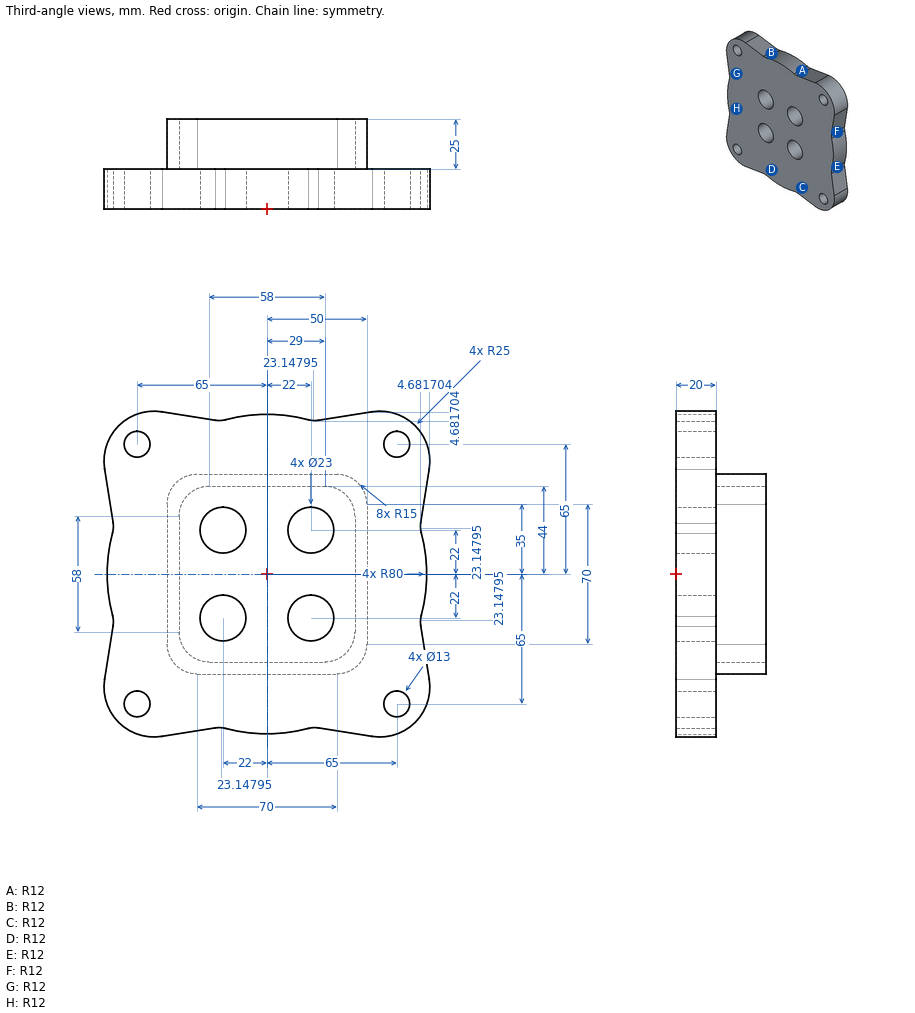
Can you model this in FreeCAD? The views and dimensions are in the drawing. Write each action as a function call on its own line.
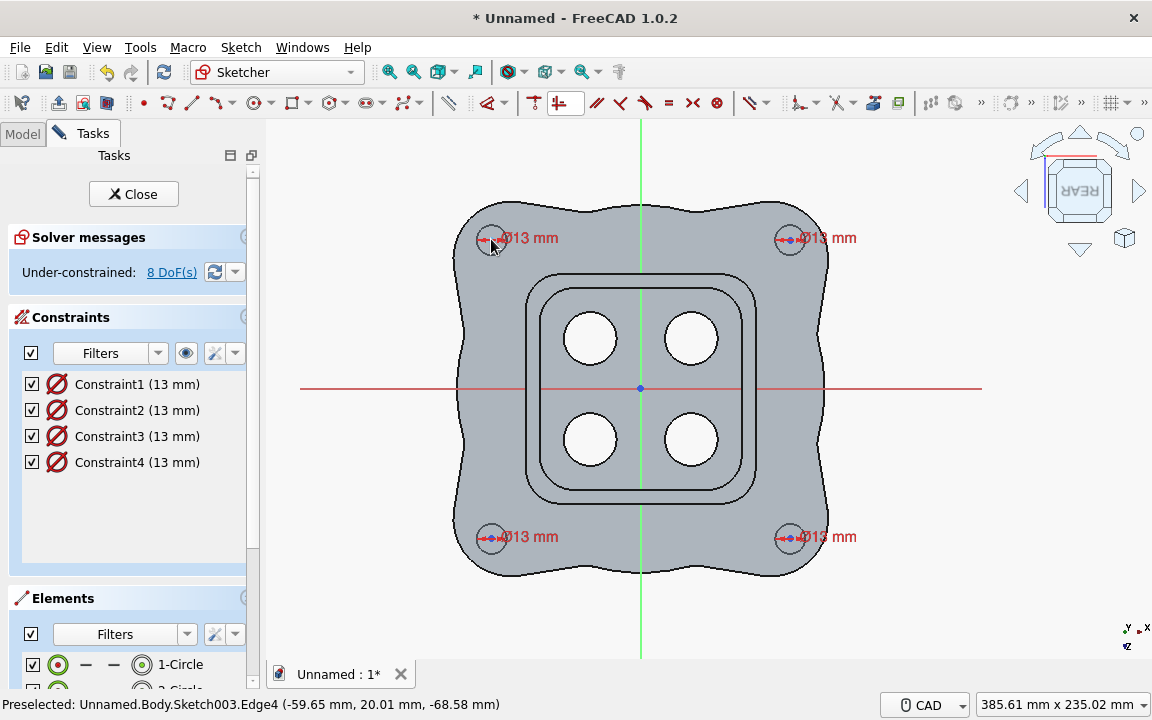
click(790, 240)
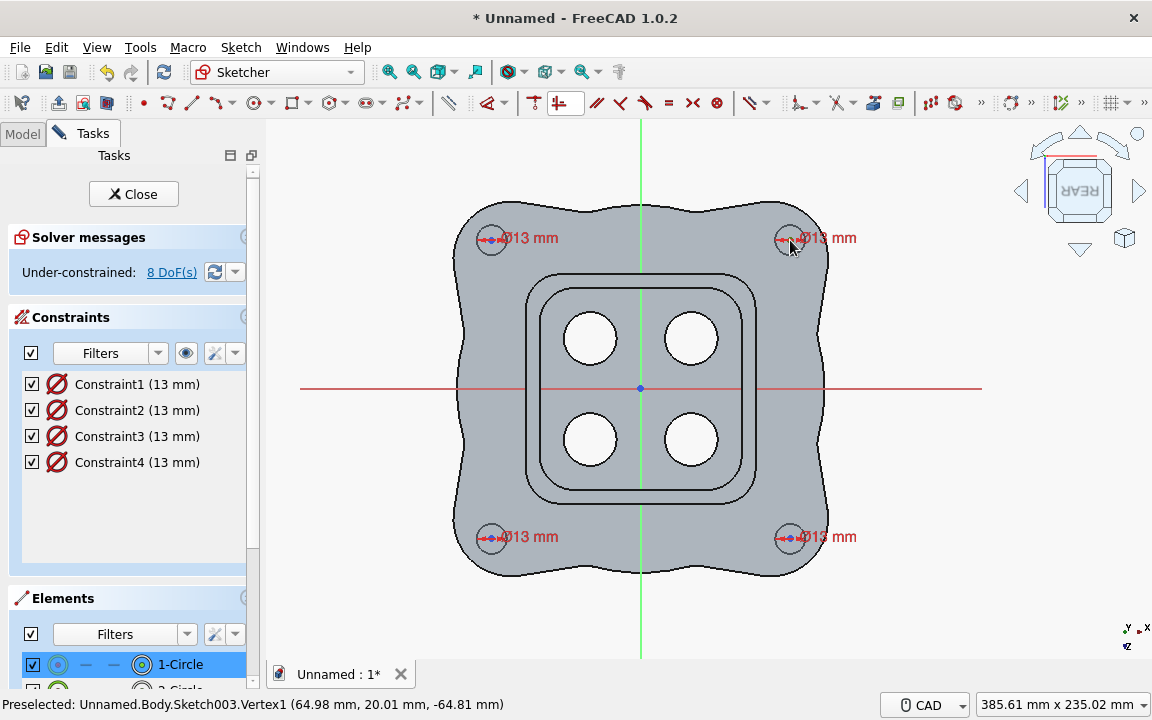
click(790, 539)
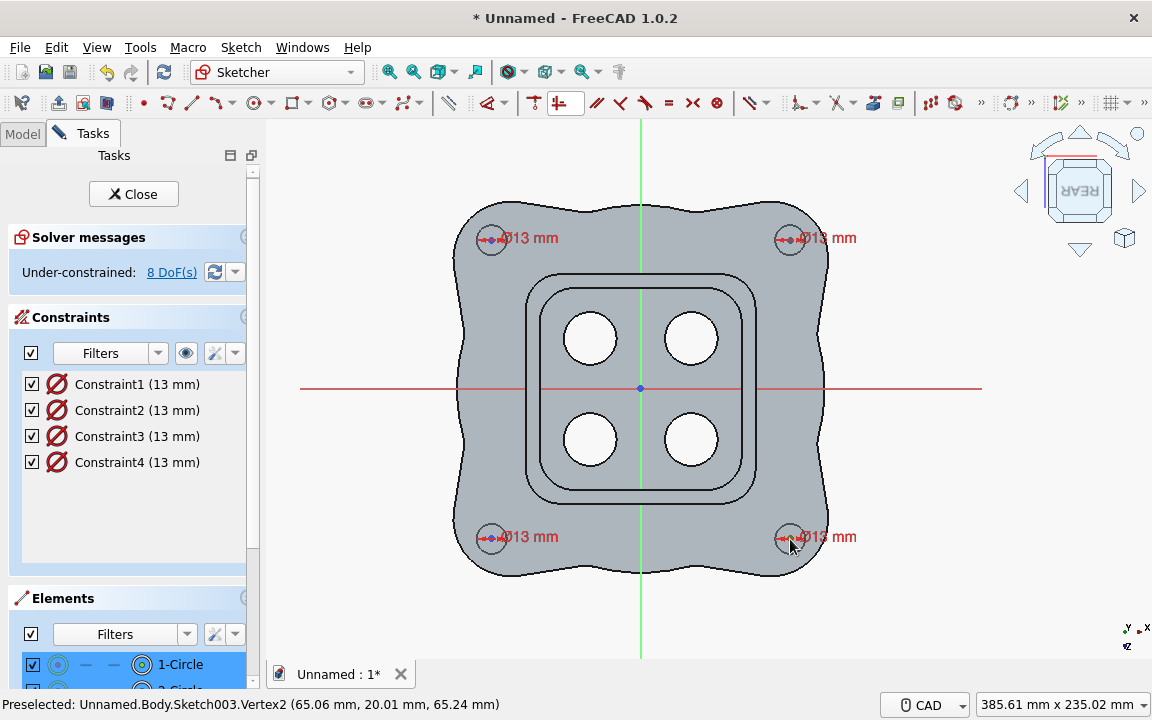
key(v)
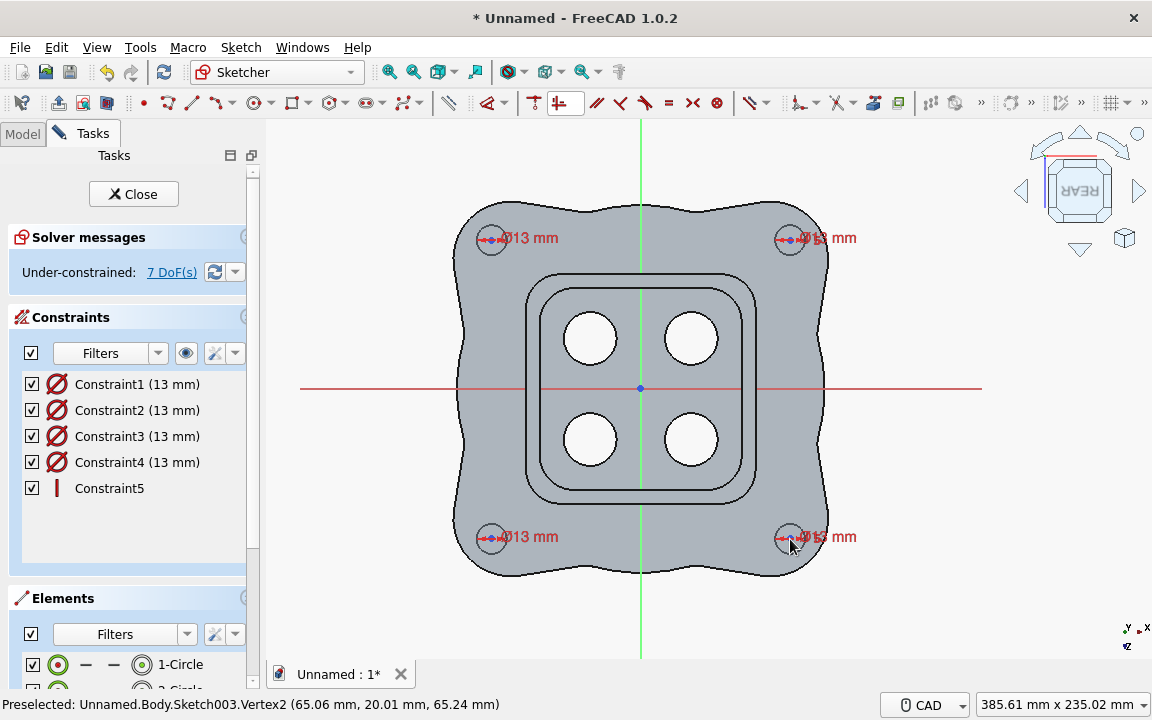
click(790, 539)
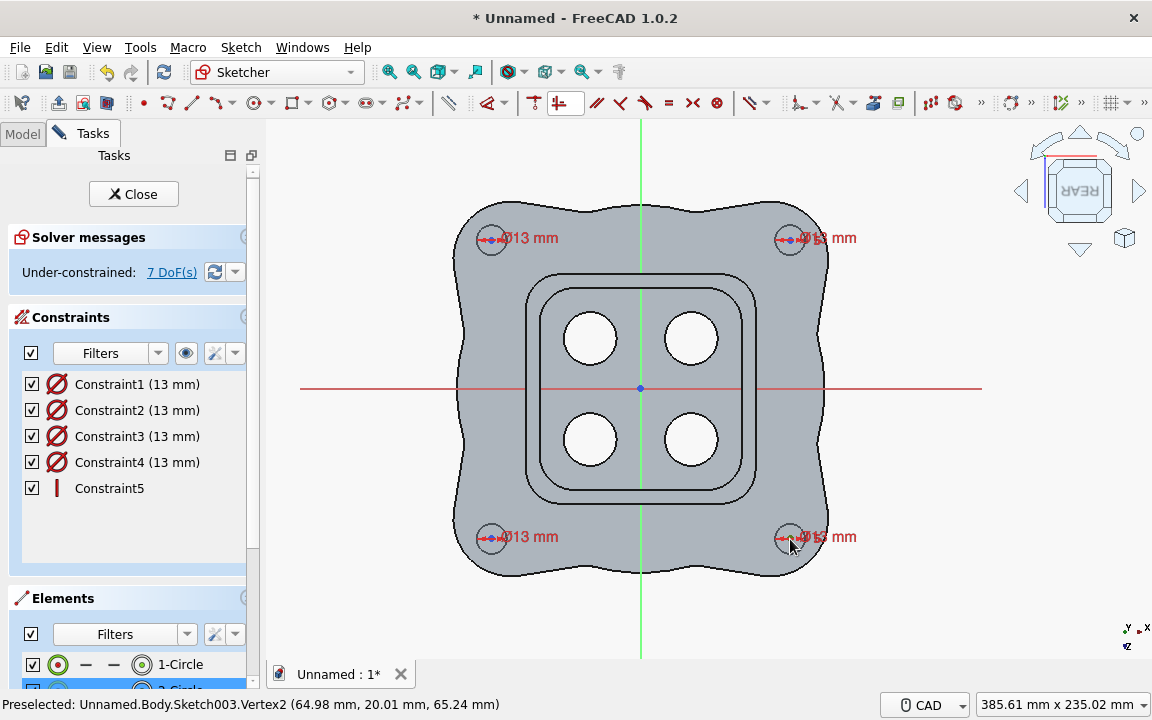
click(492, 539)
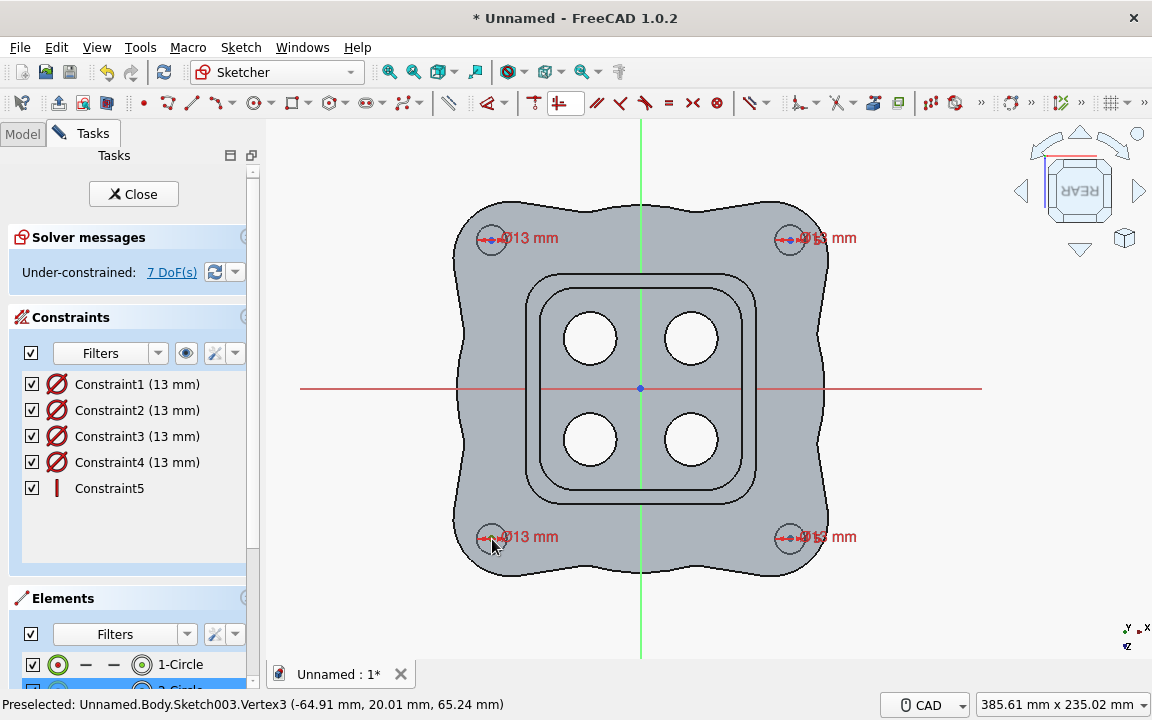
click(578, 104)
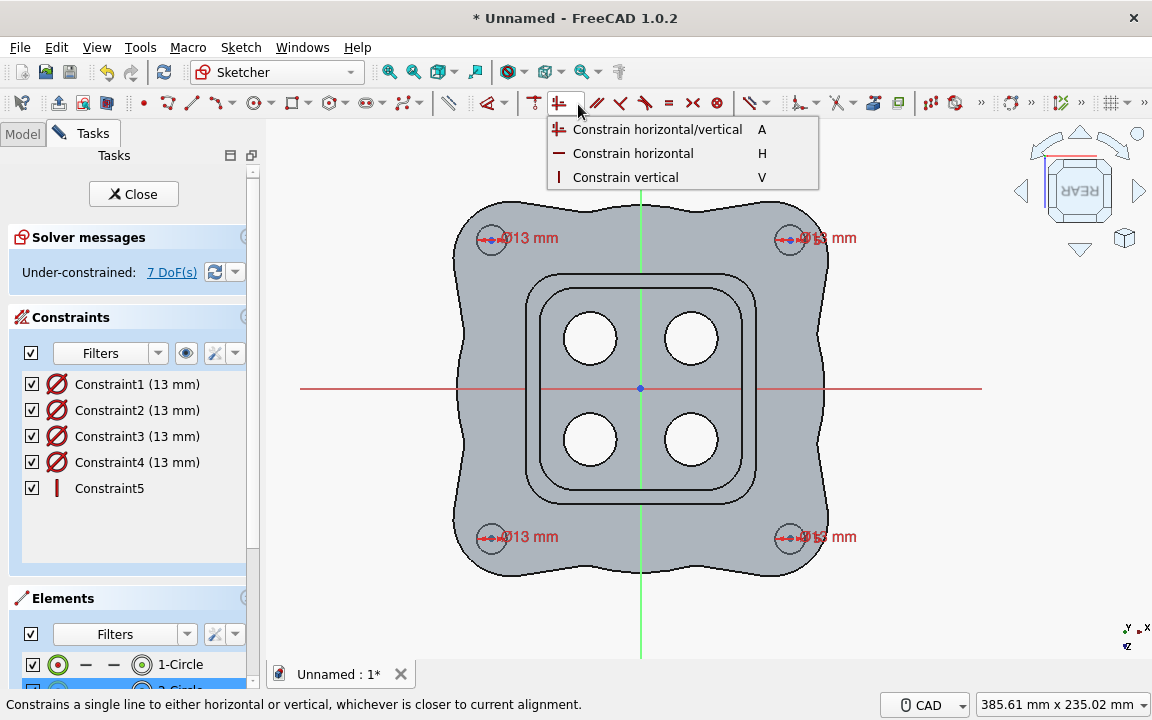
click(683, 153)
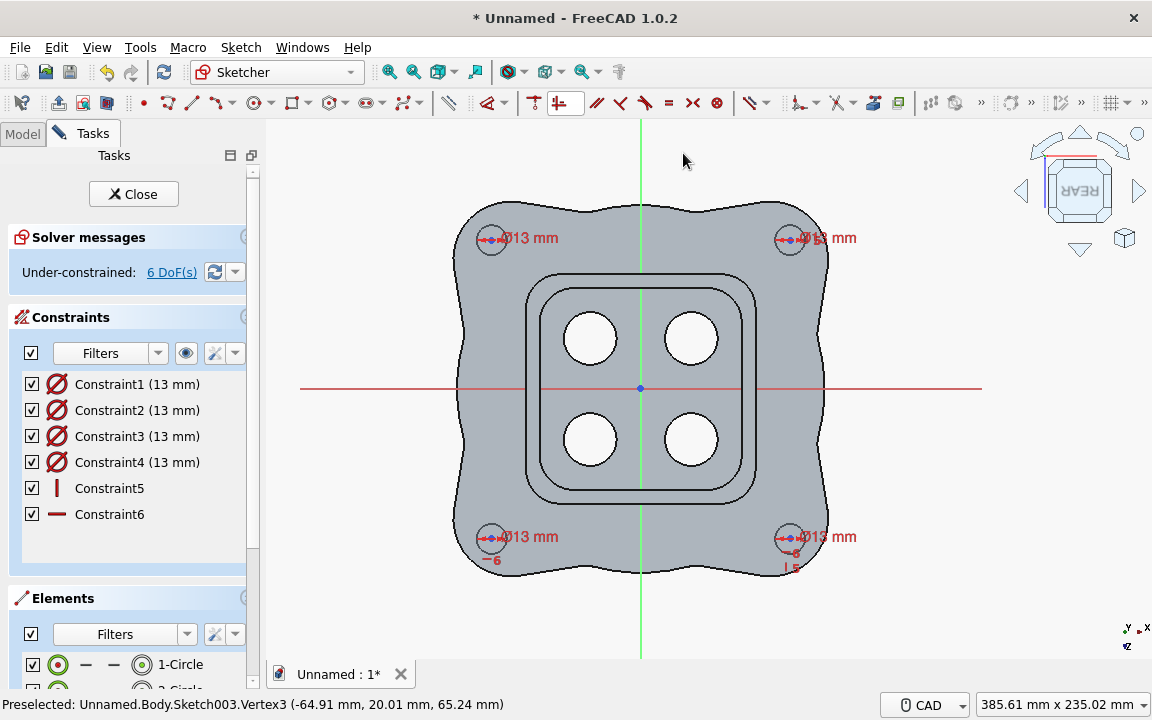
click(492, 539)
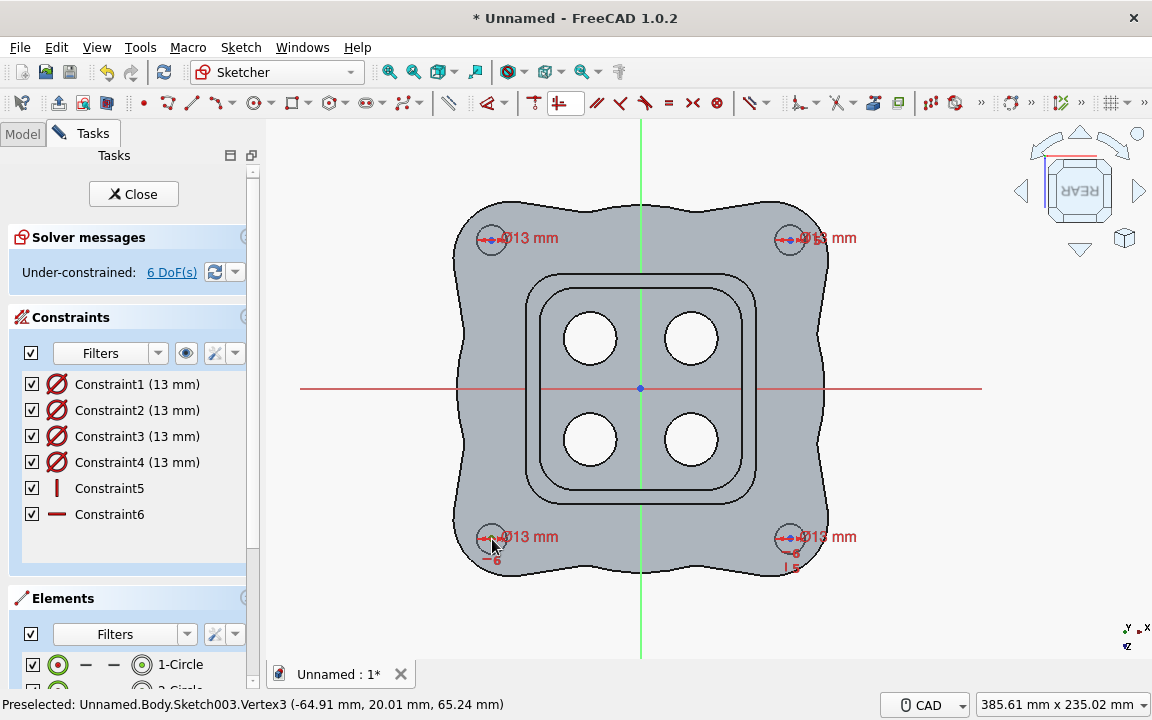
click(492, 240)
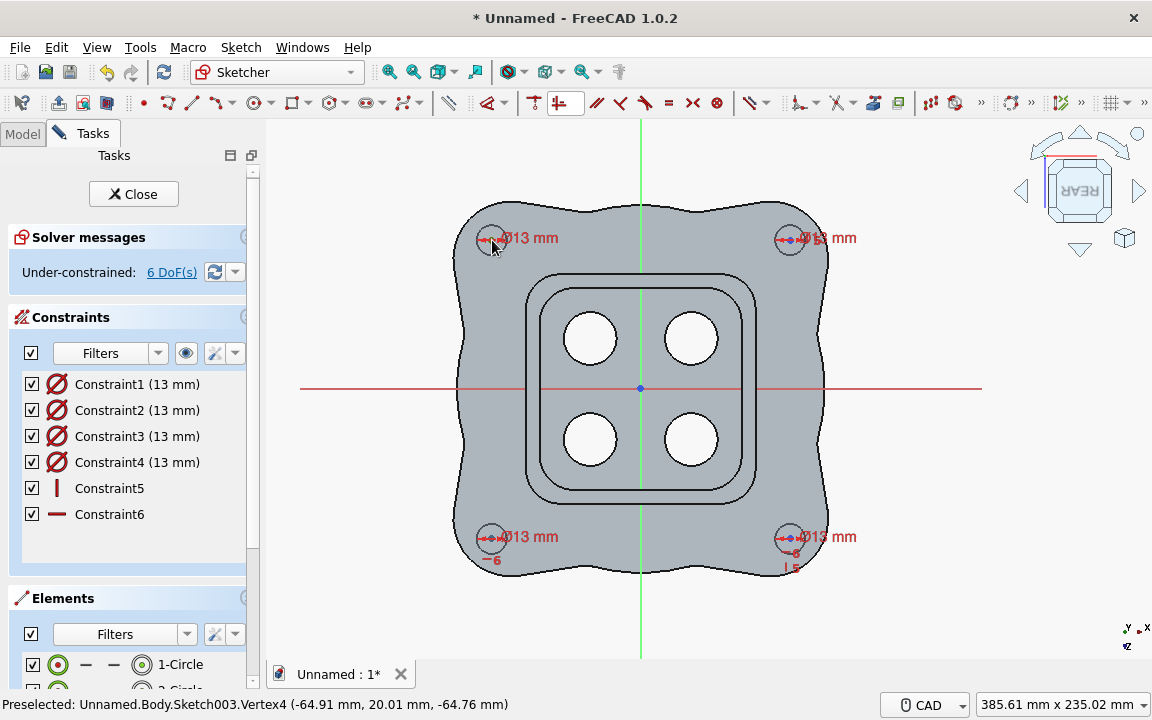
click(578, 104)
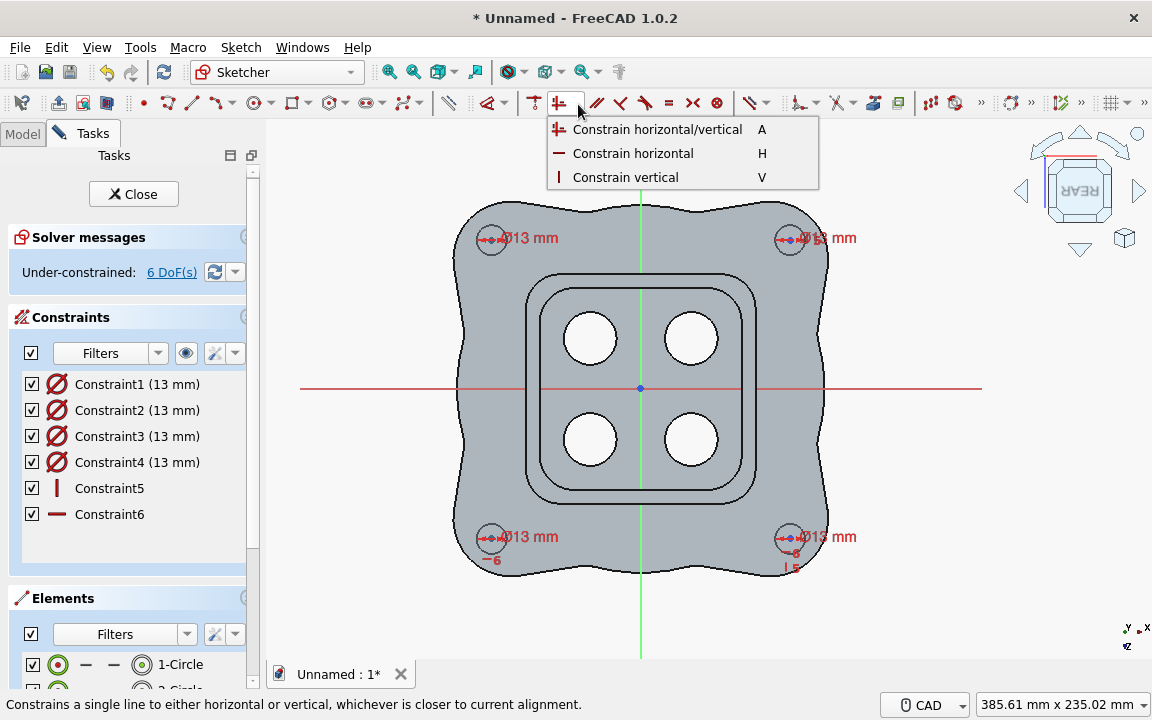
click(683, 177)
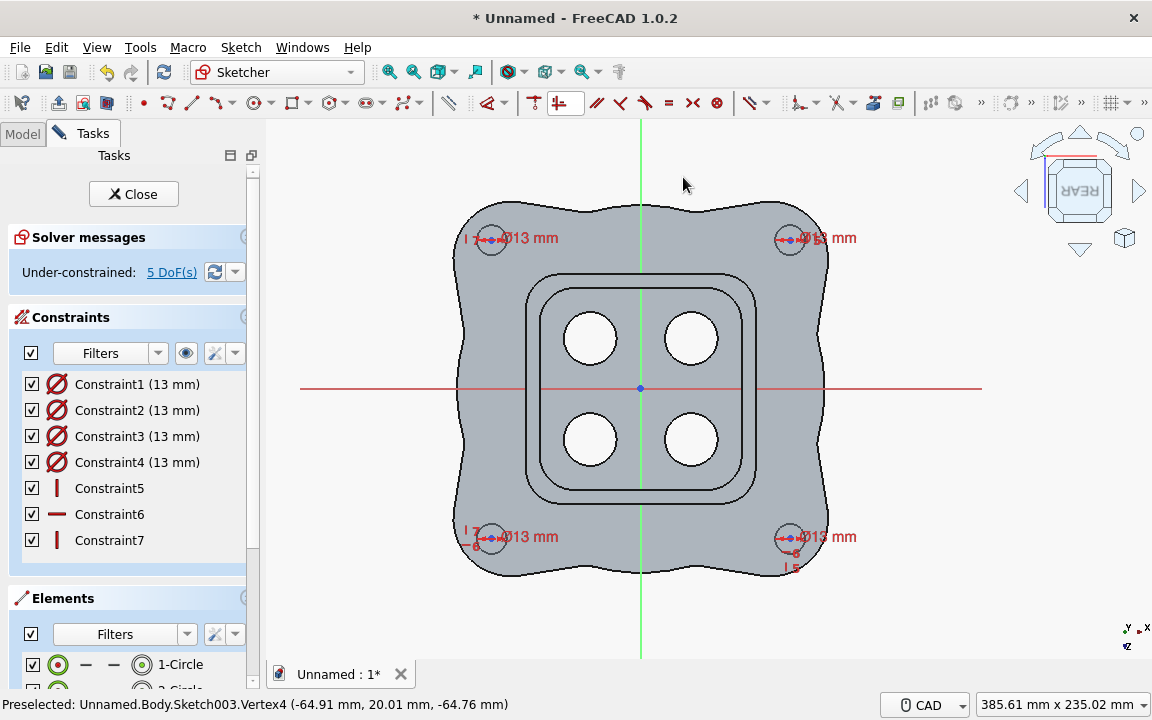
click(790, 240)